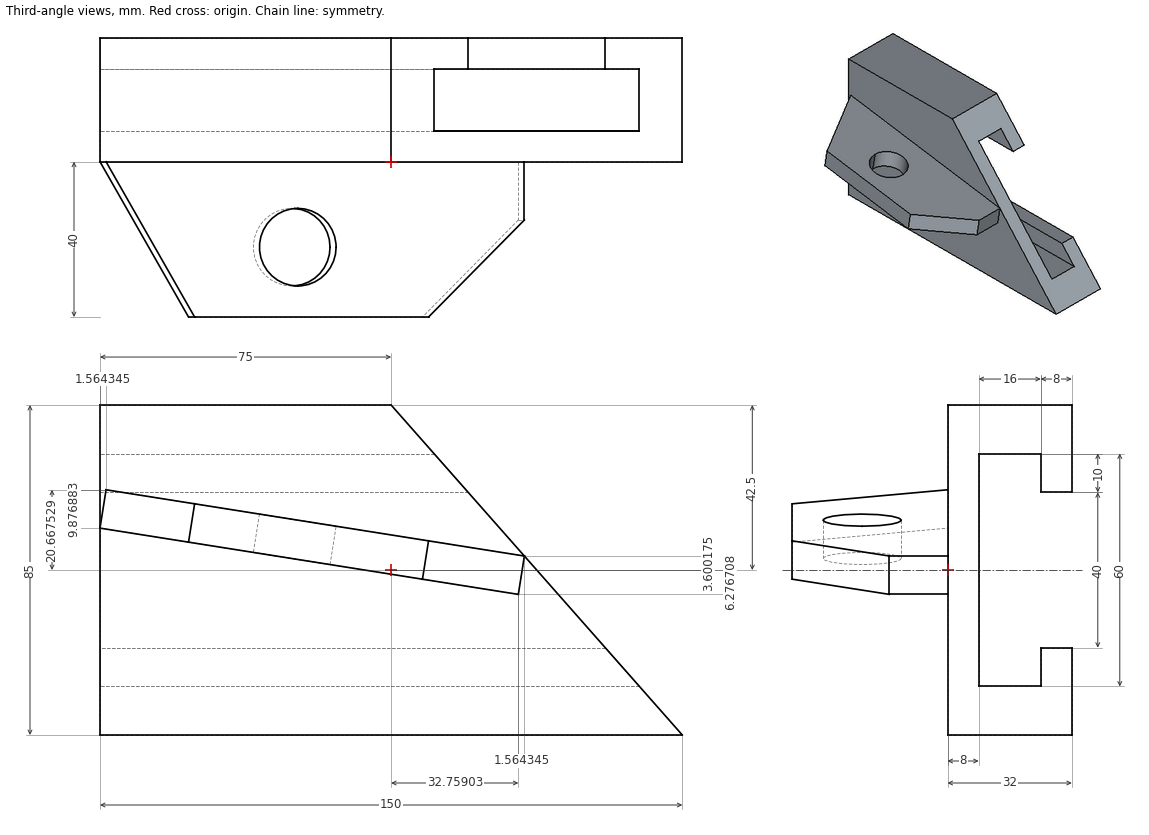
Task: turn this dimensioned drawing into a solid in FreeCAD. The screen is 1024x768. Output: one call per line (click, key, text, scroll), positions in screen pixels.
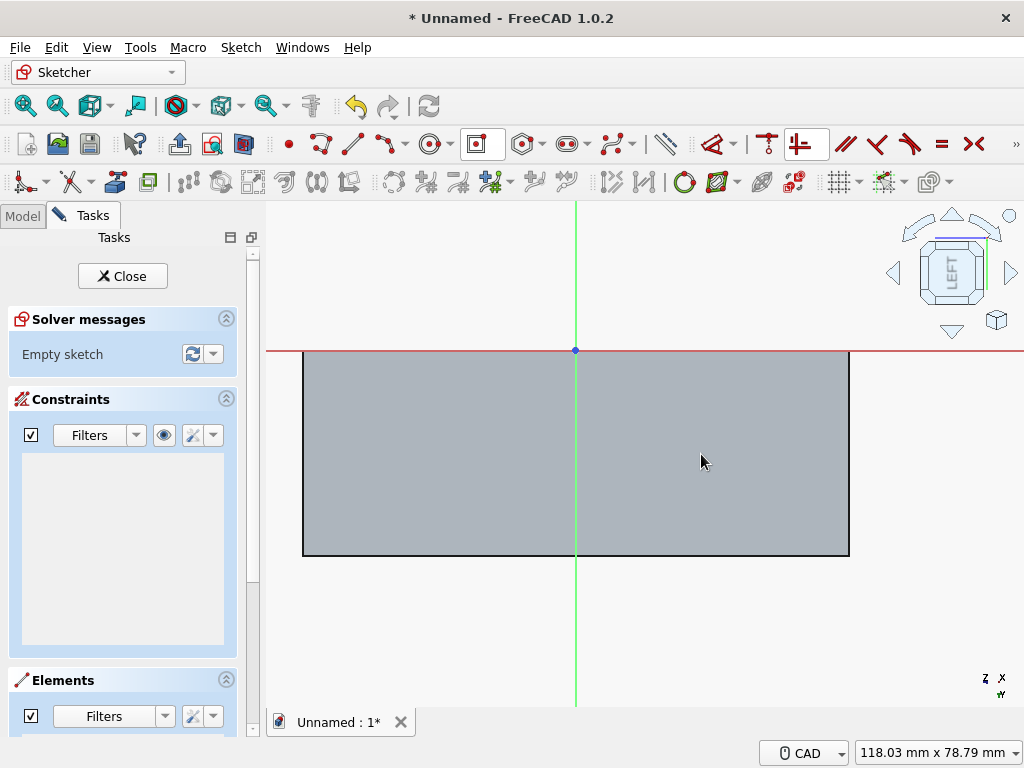
key(g)
key(m)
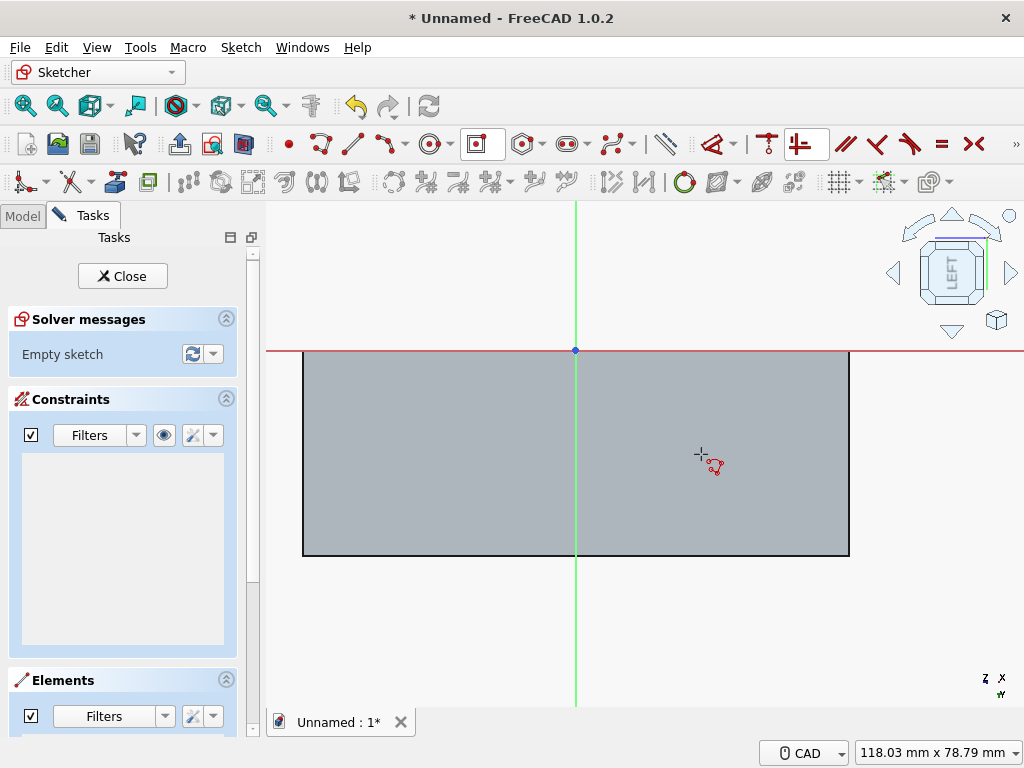
click(768, 402)
click(383, 402)
click(383, 505)
click(447, 505)
click(447, 556)
click(704, 556)
click(704, 505)
click(768, 505)
click(768, 403)
key(Escape)
key(Escape)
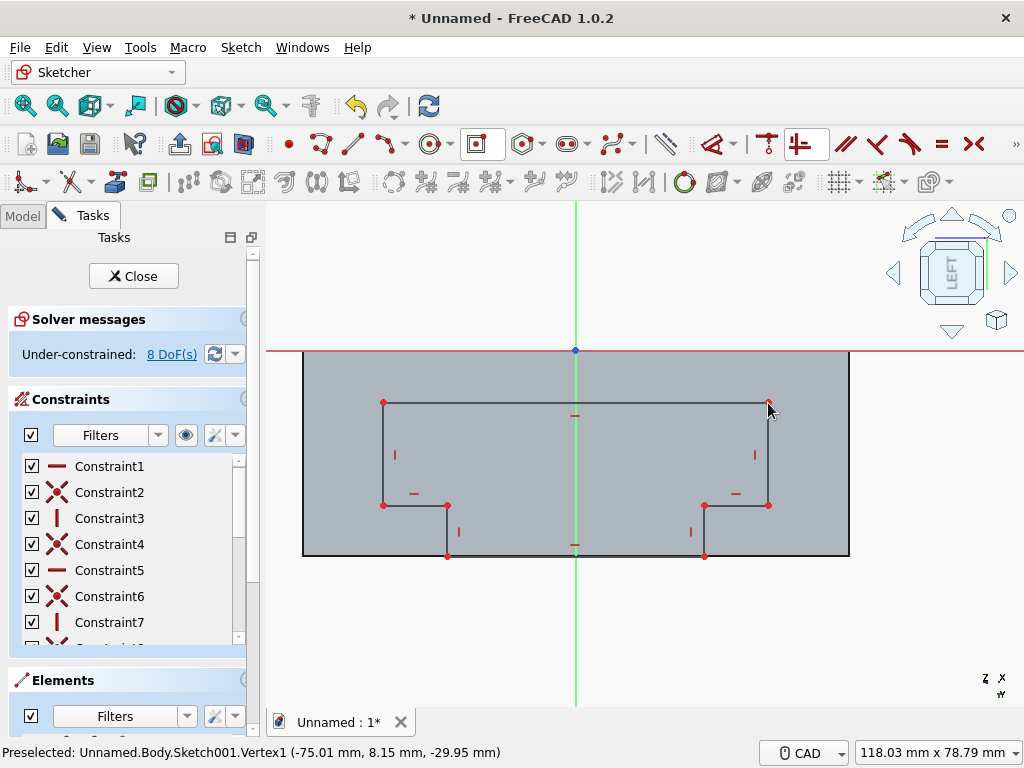
click(447, 506)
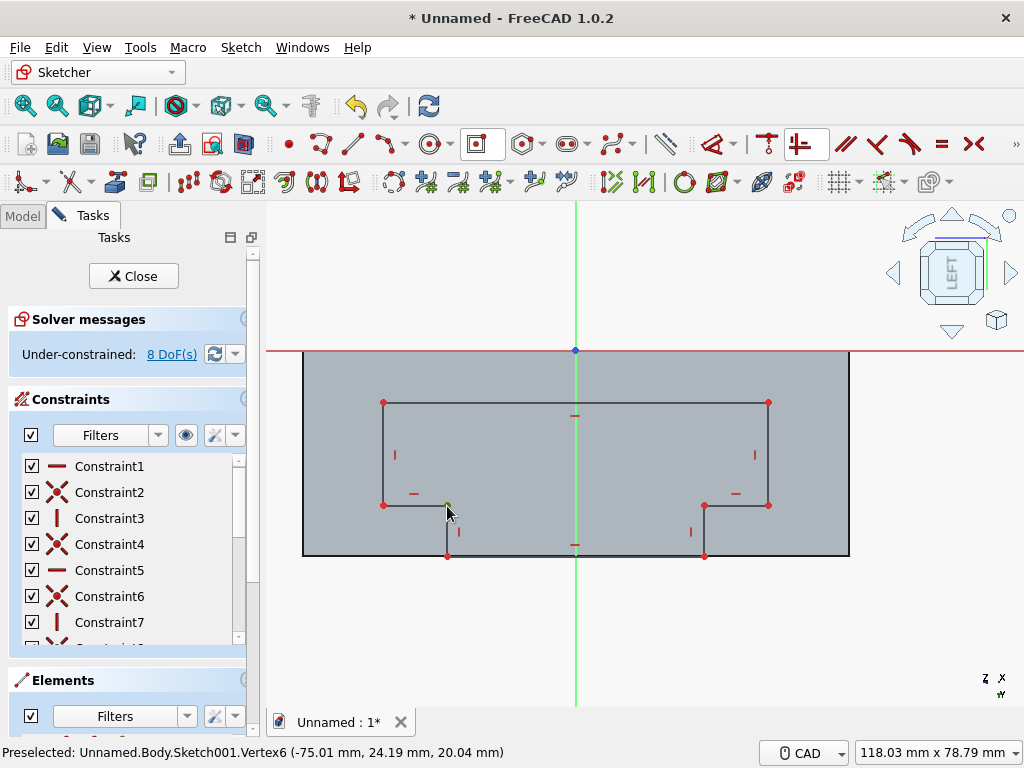
click(704, 506)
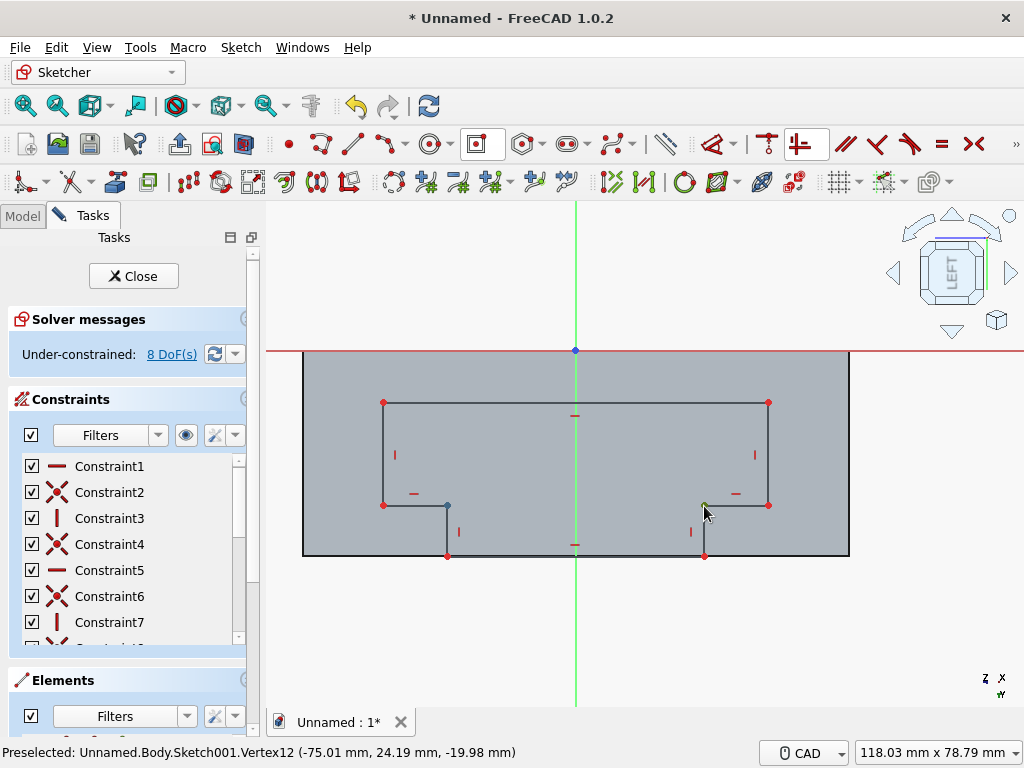
click(576, 647)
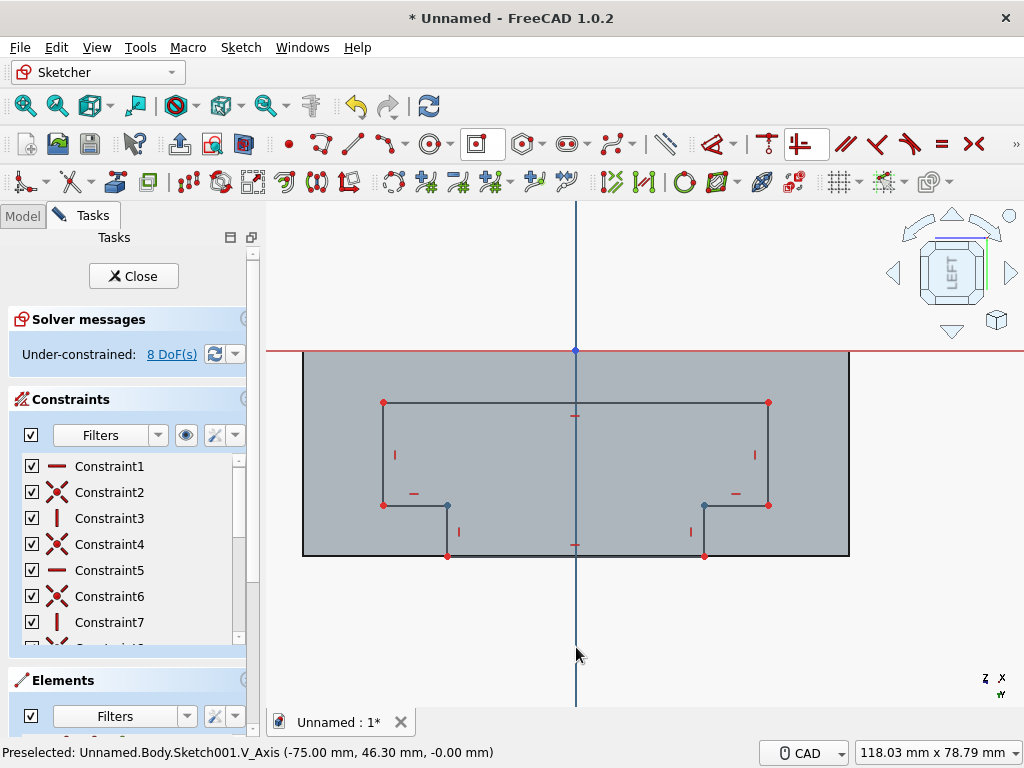
key(s)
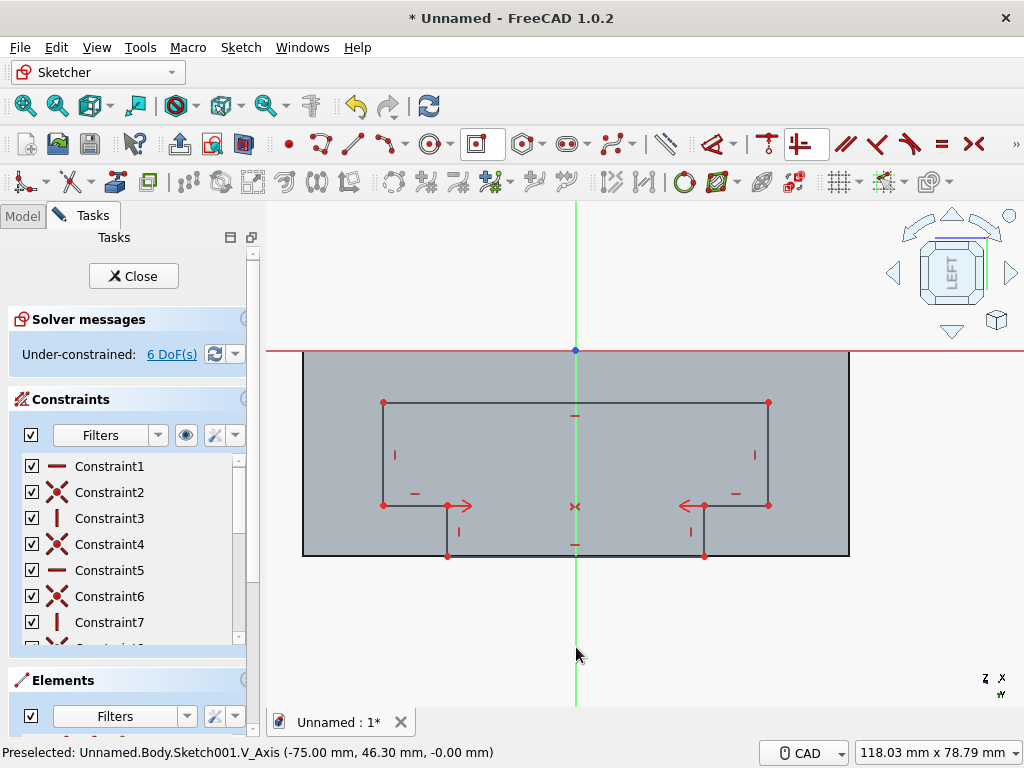
key(d)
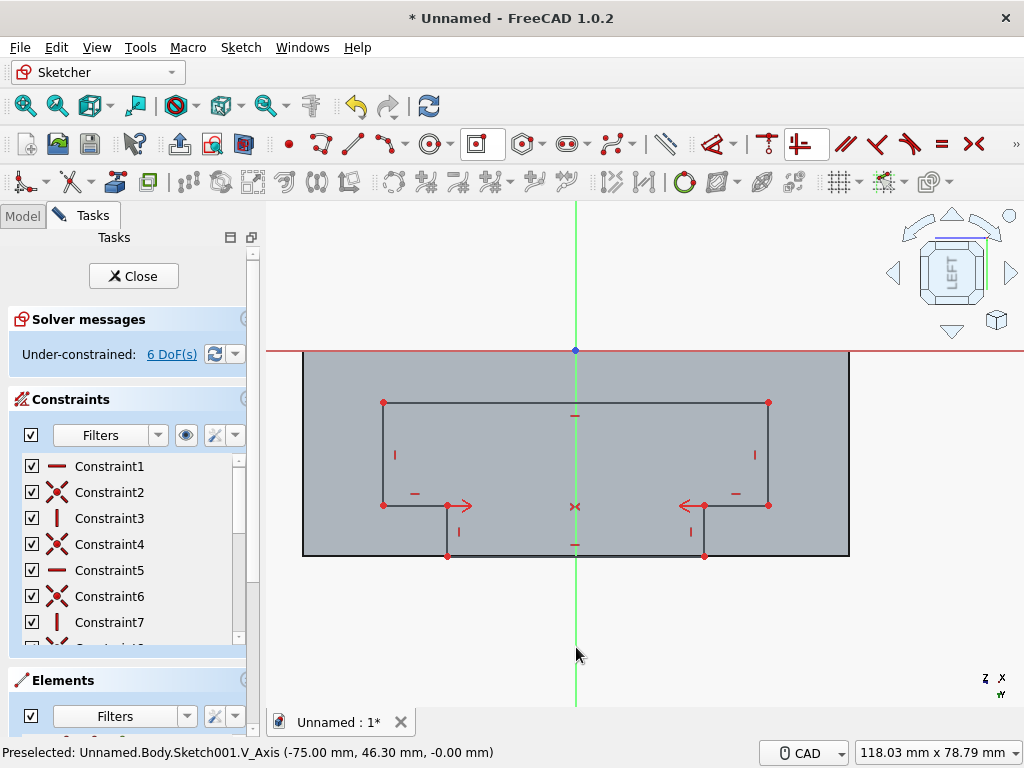
click(447, 521)
click(413, 532)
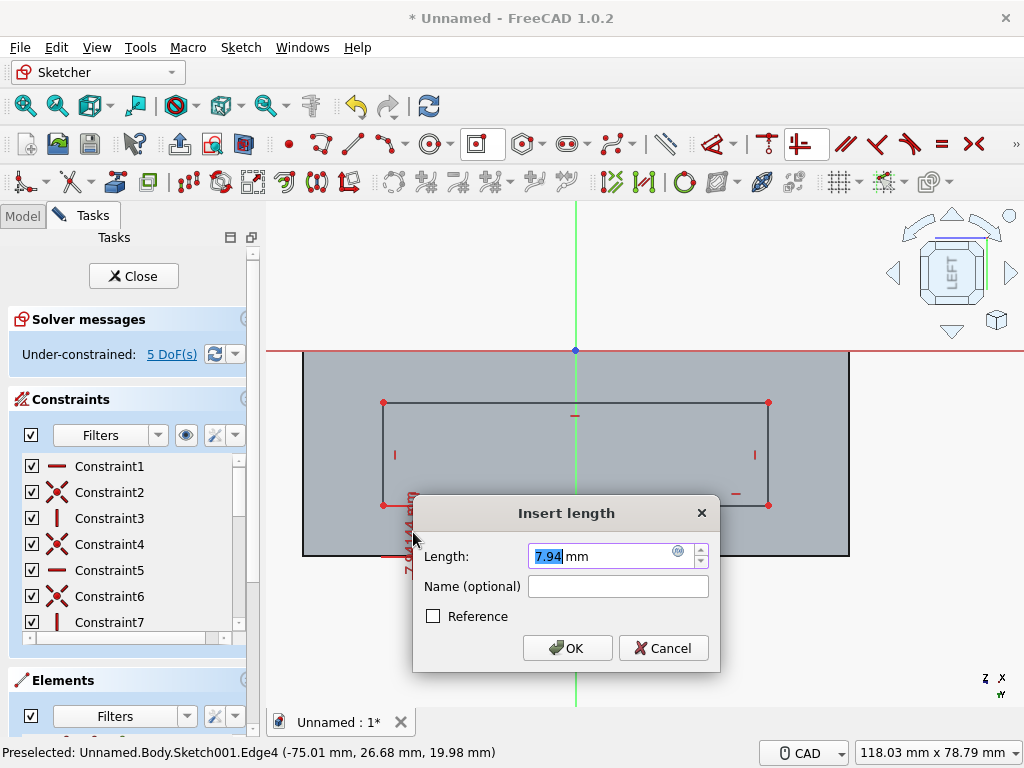
text(8)
key(Return)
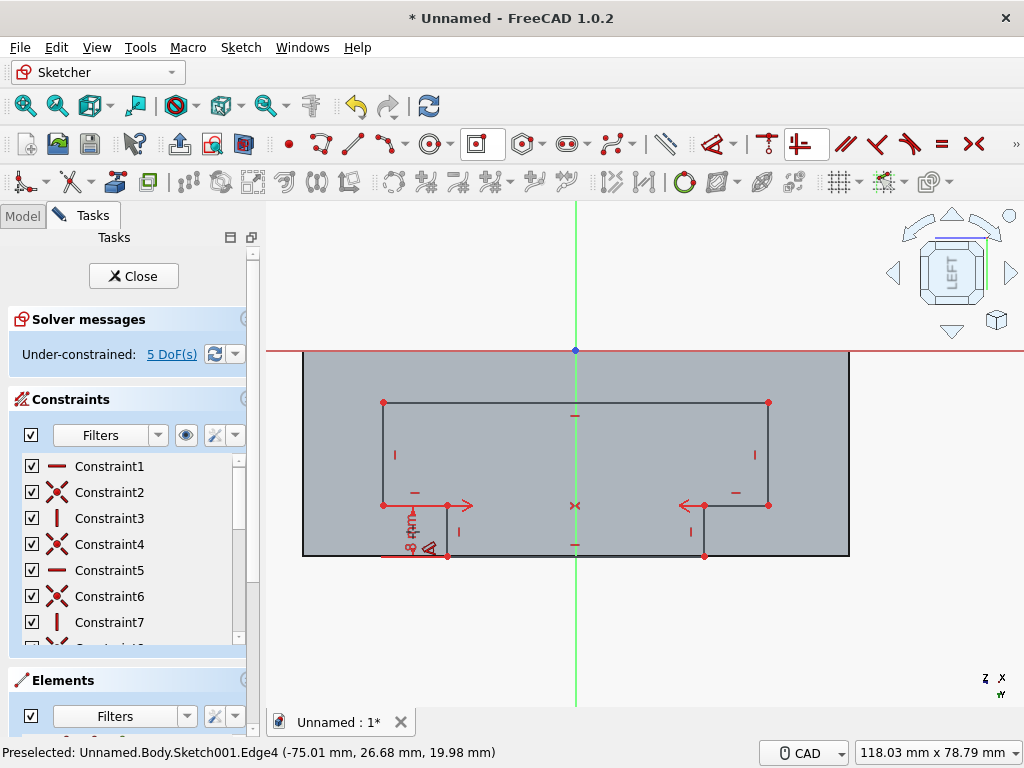
click(652, 403)
click(487, 369)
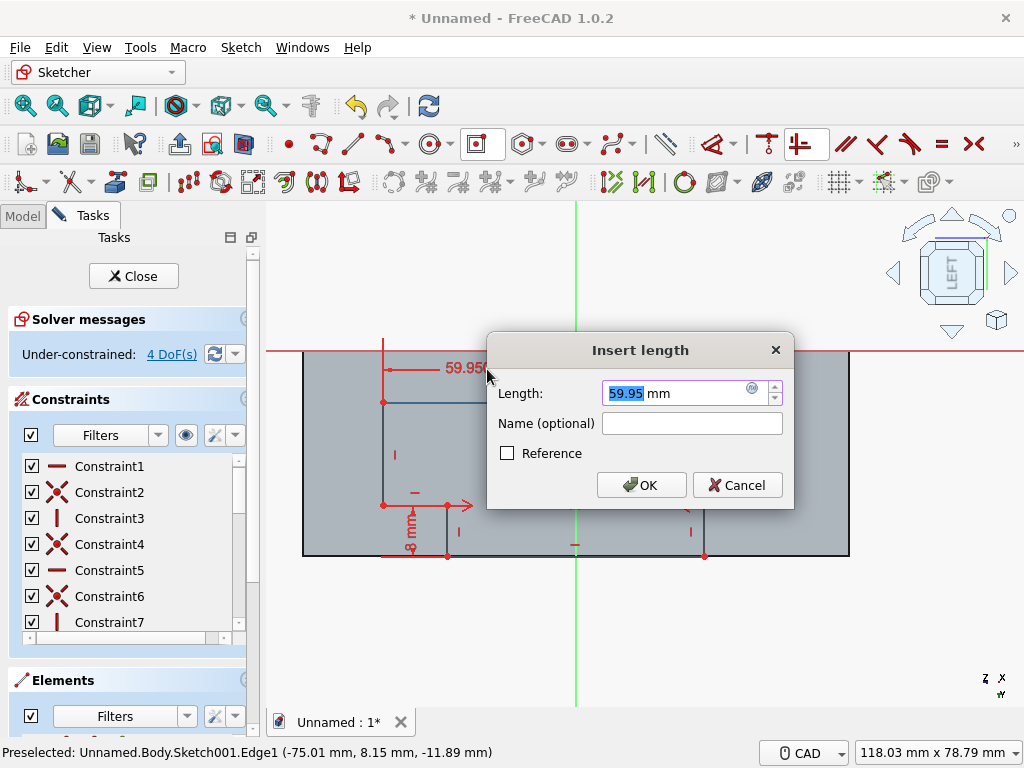
text(60)
key(Return)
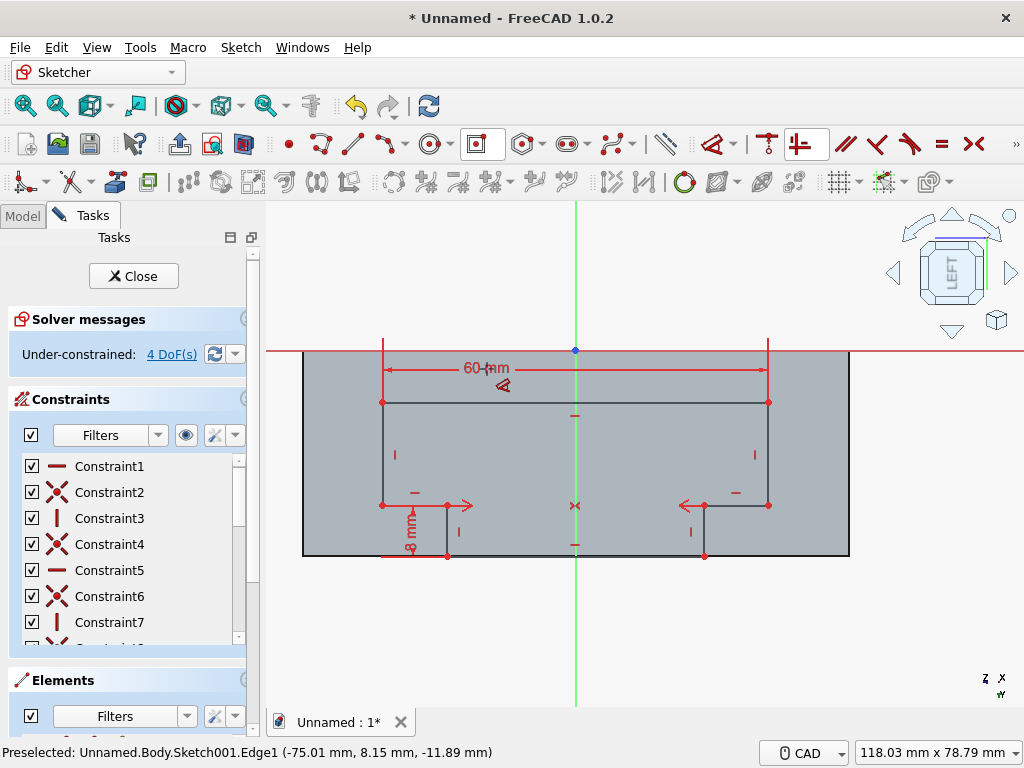
click(383, 434)
click(349, 454)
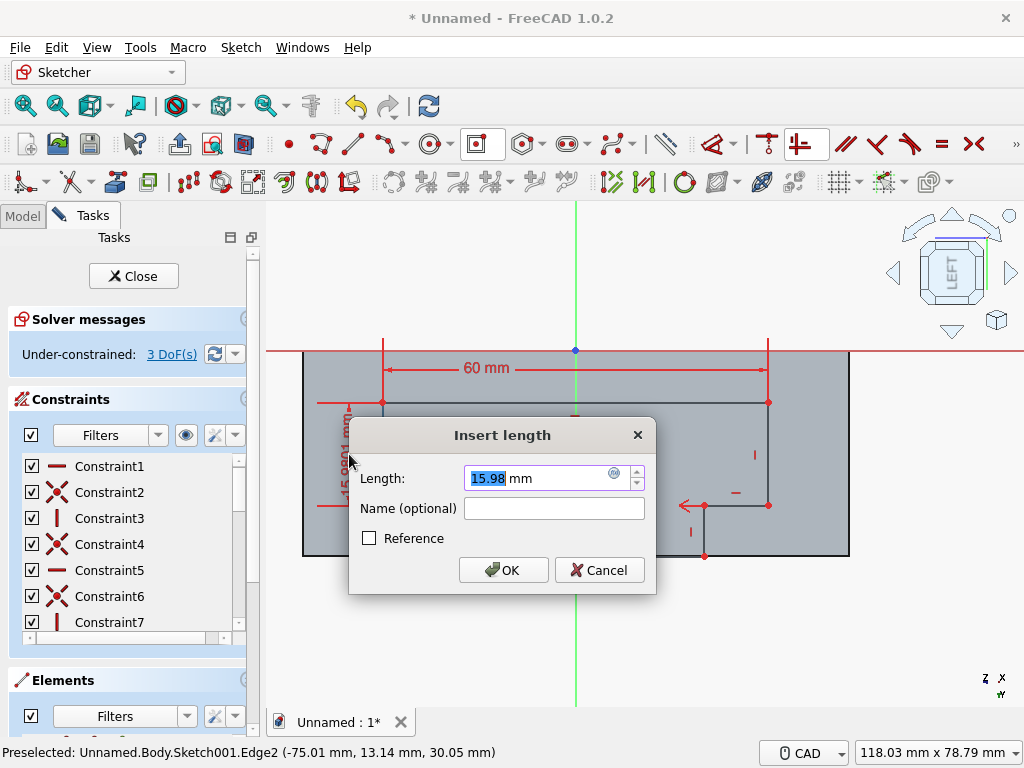
text(16)
key(Return)